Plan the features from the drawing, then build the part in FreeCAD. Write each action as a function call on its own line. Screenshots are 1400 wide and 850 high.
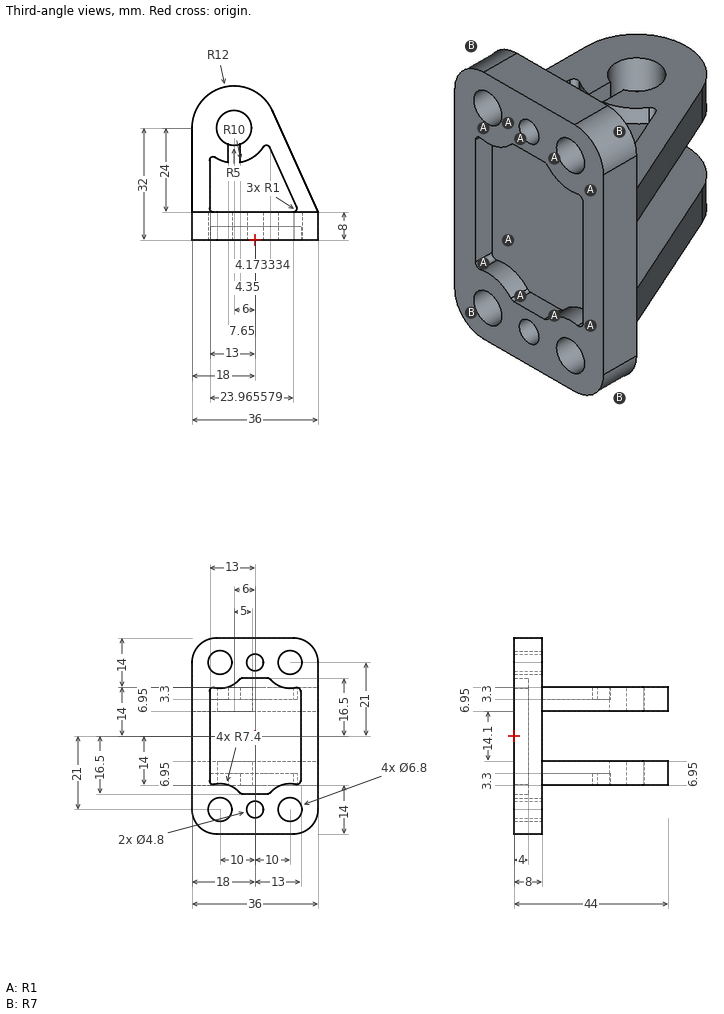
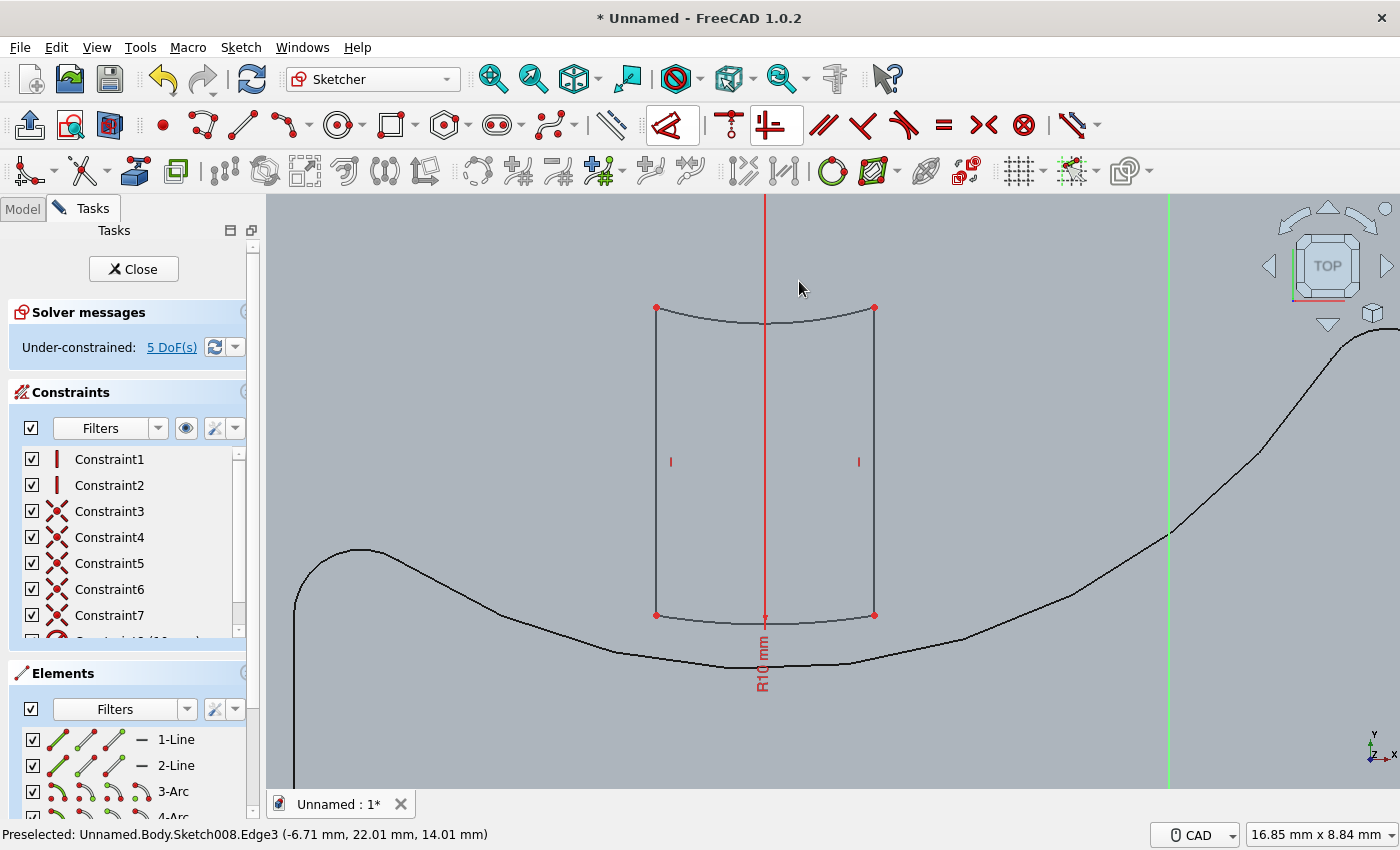
click(721, 321)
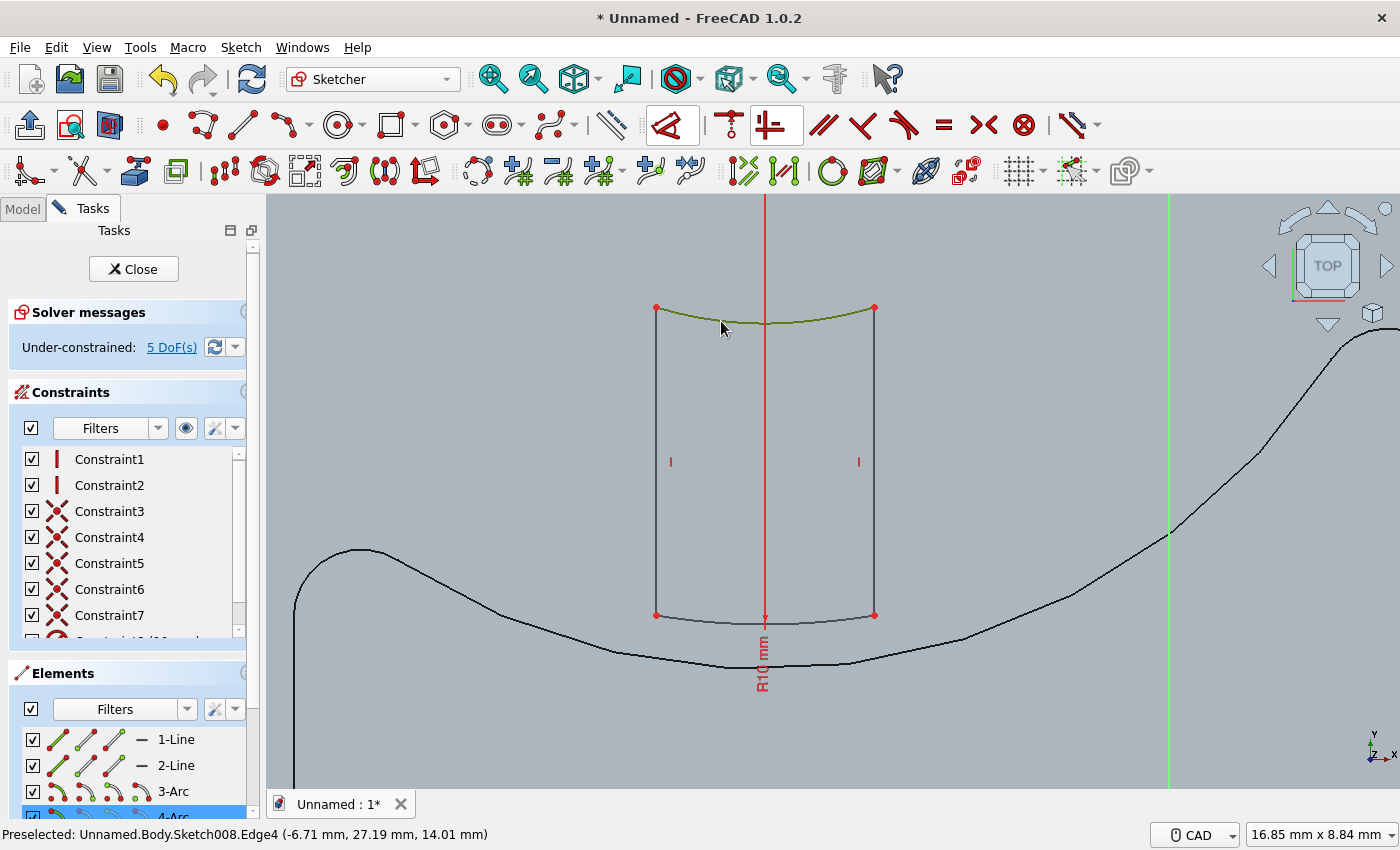
key(k)
key(r)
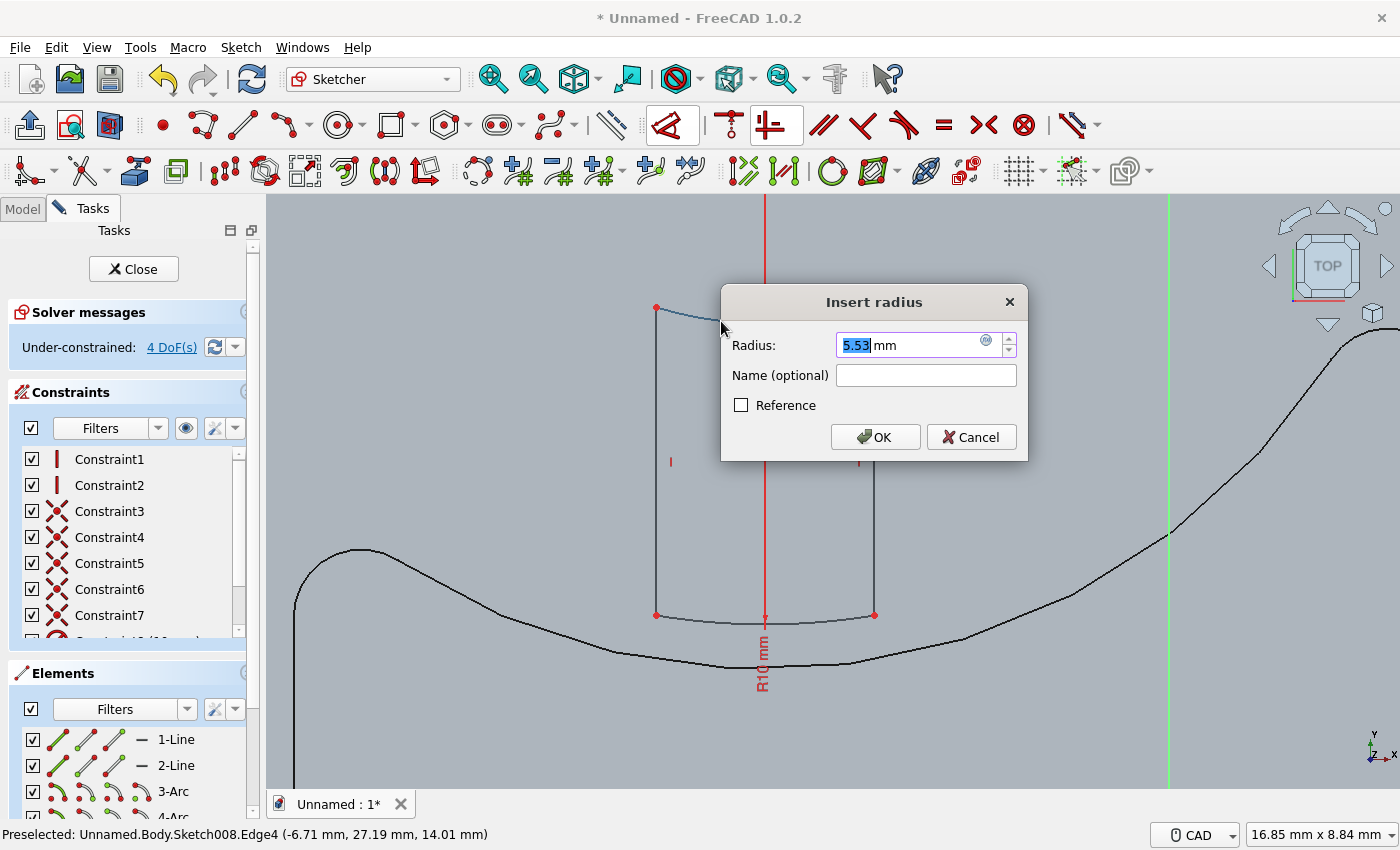
text(5)
key(Return)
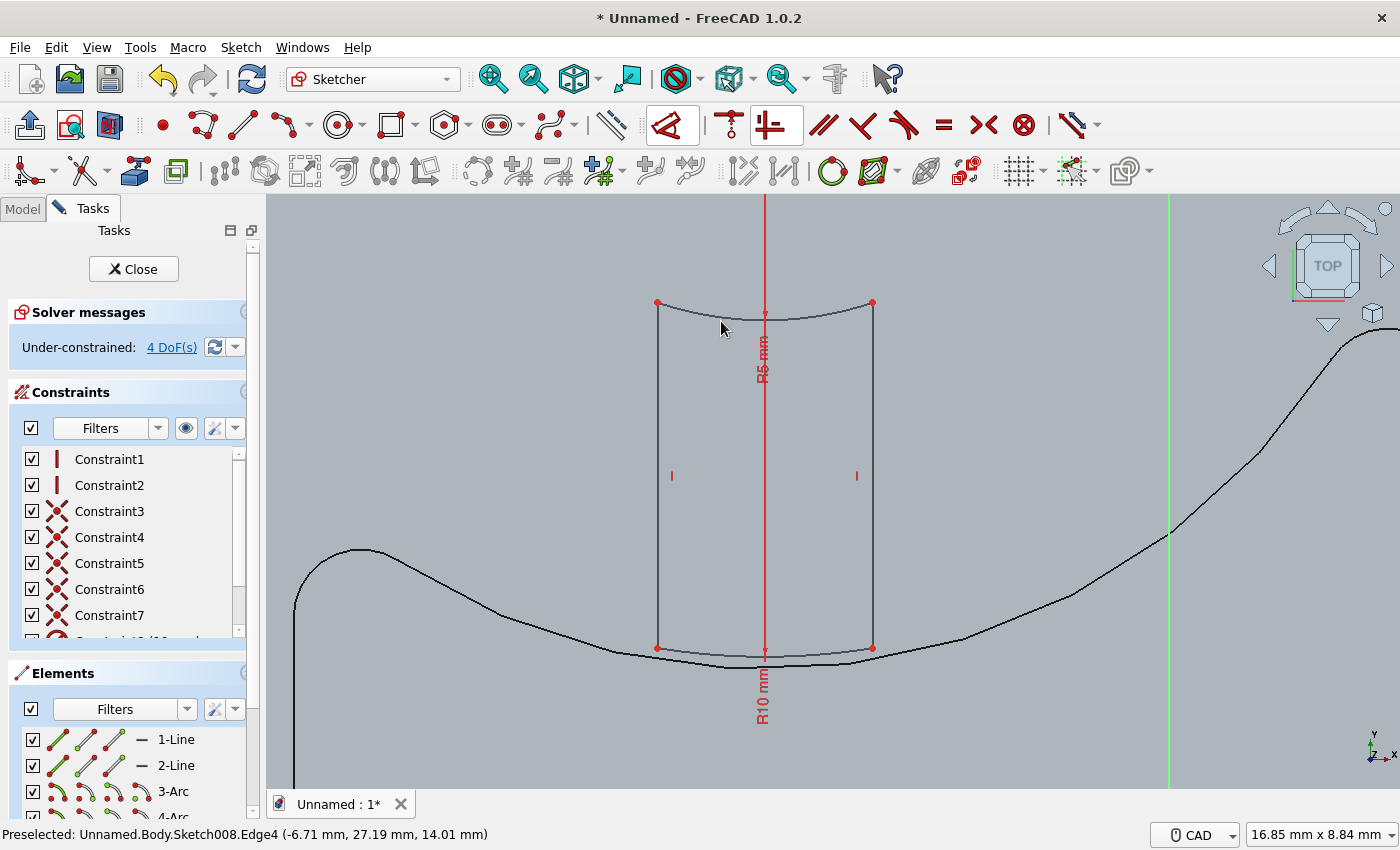
scroll(764, 692, down, 3)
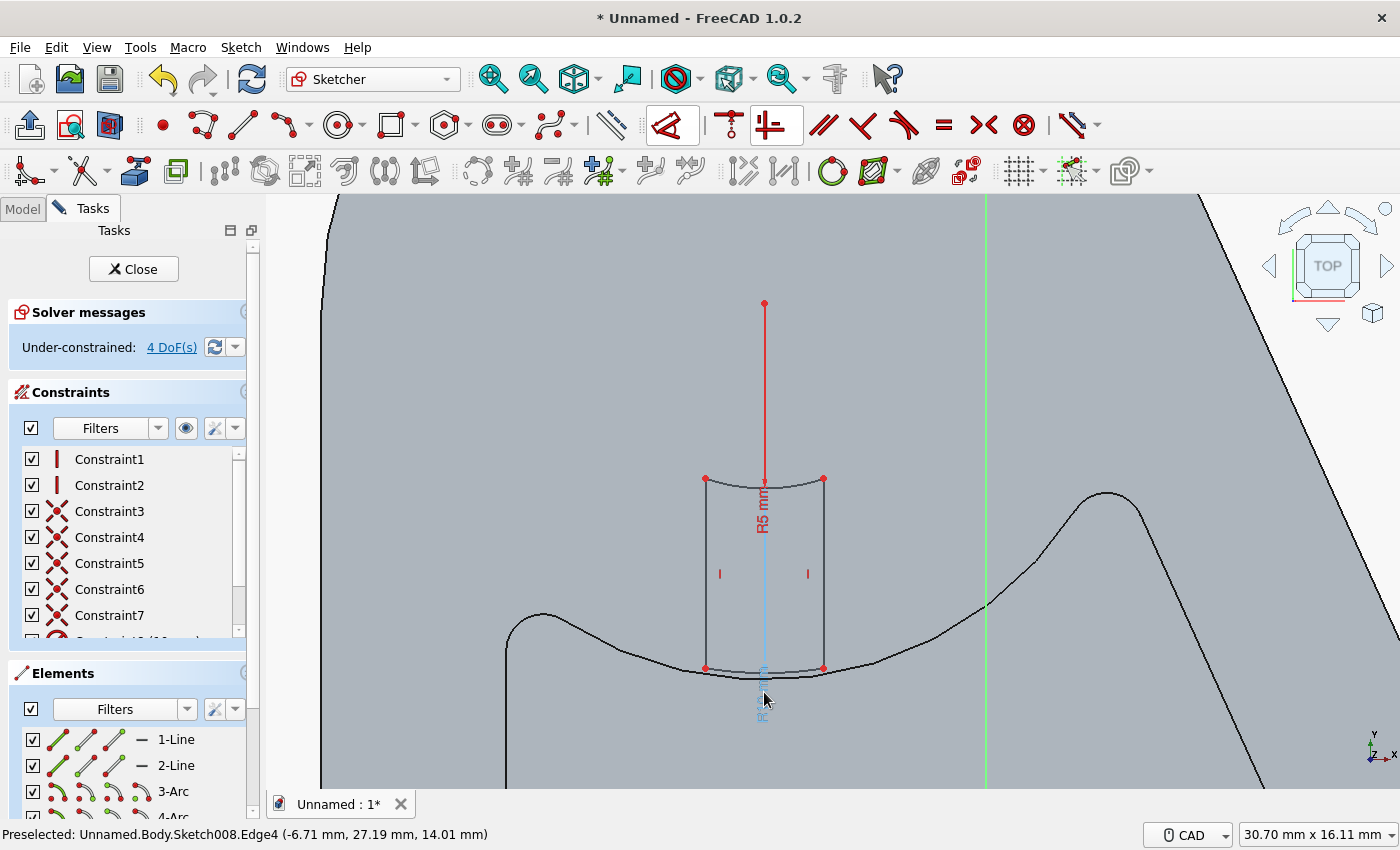
click(765, 304)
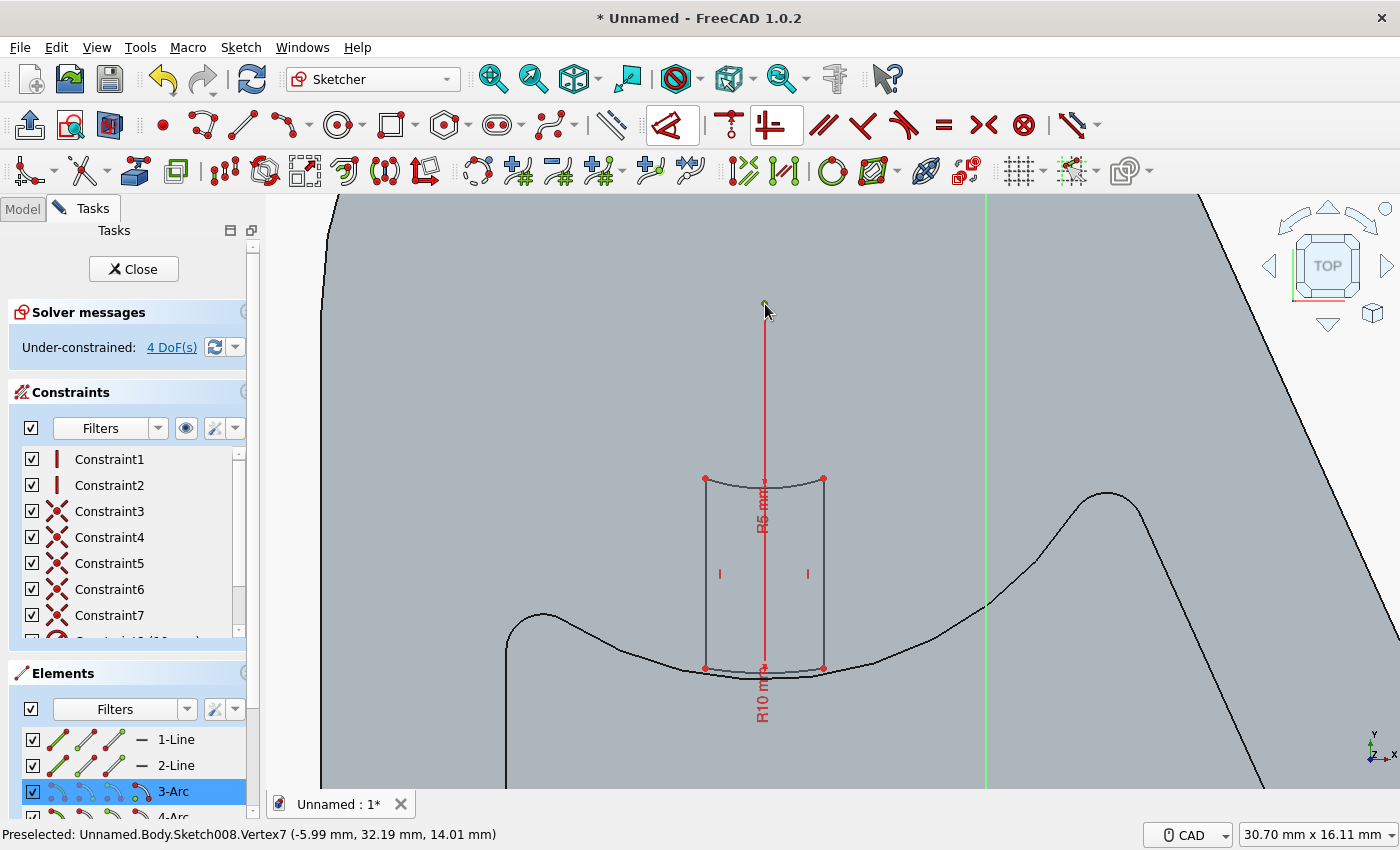
key(l)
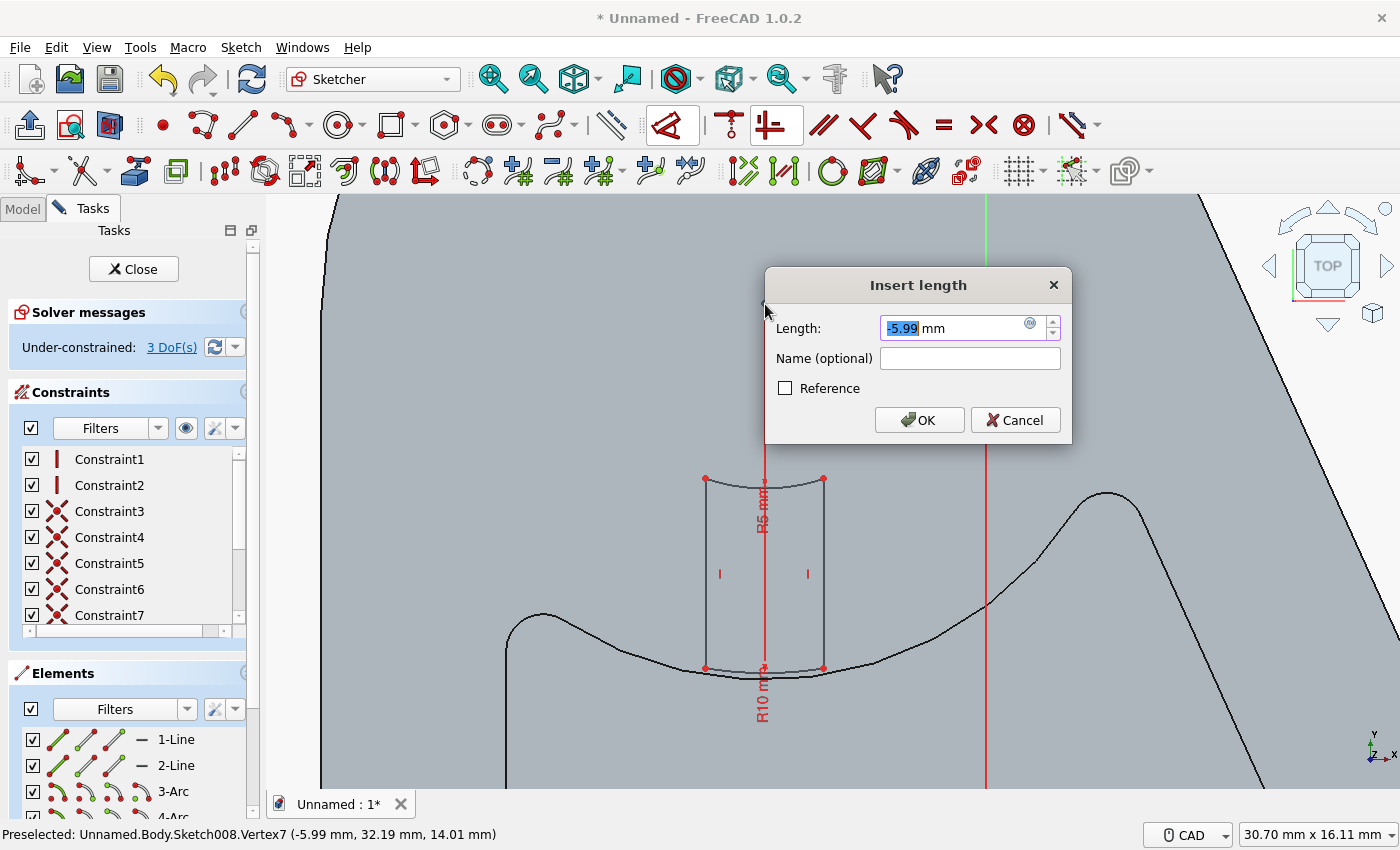
text(-6)
key(Return)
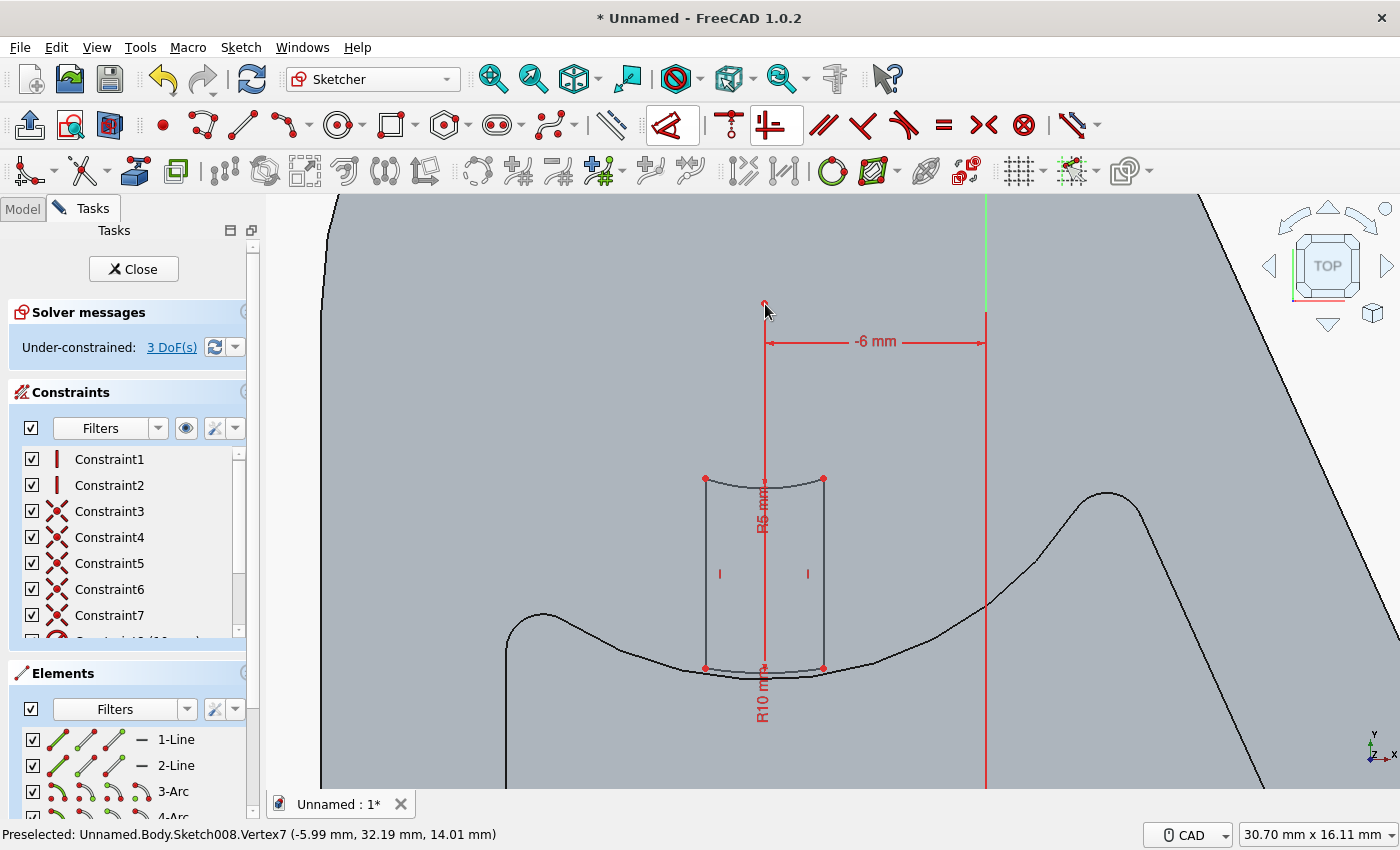
click(765, 304)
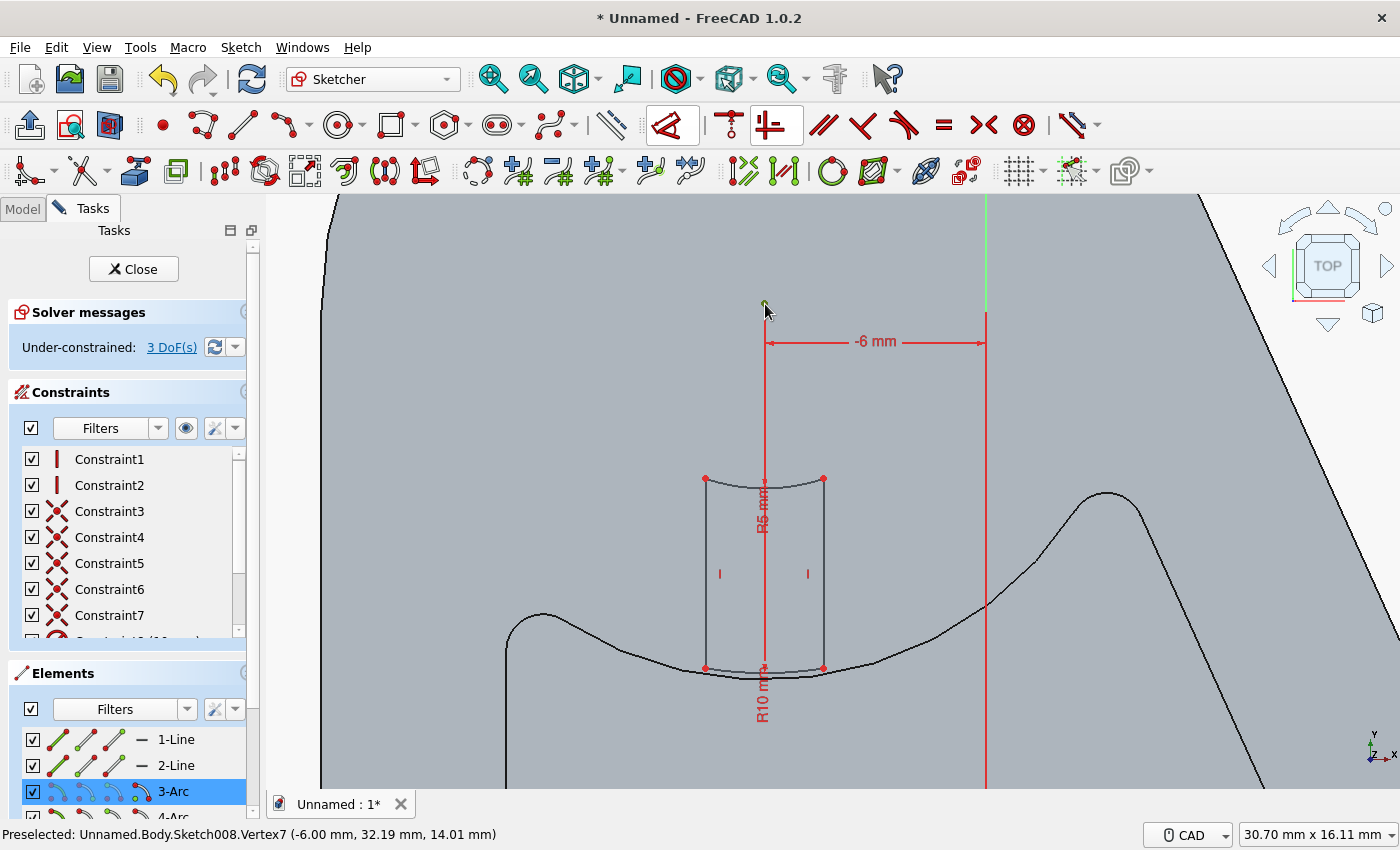
click(694, 126)